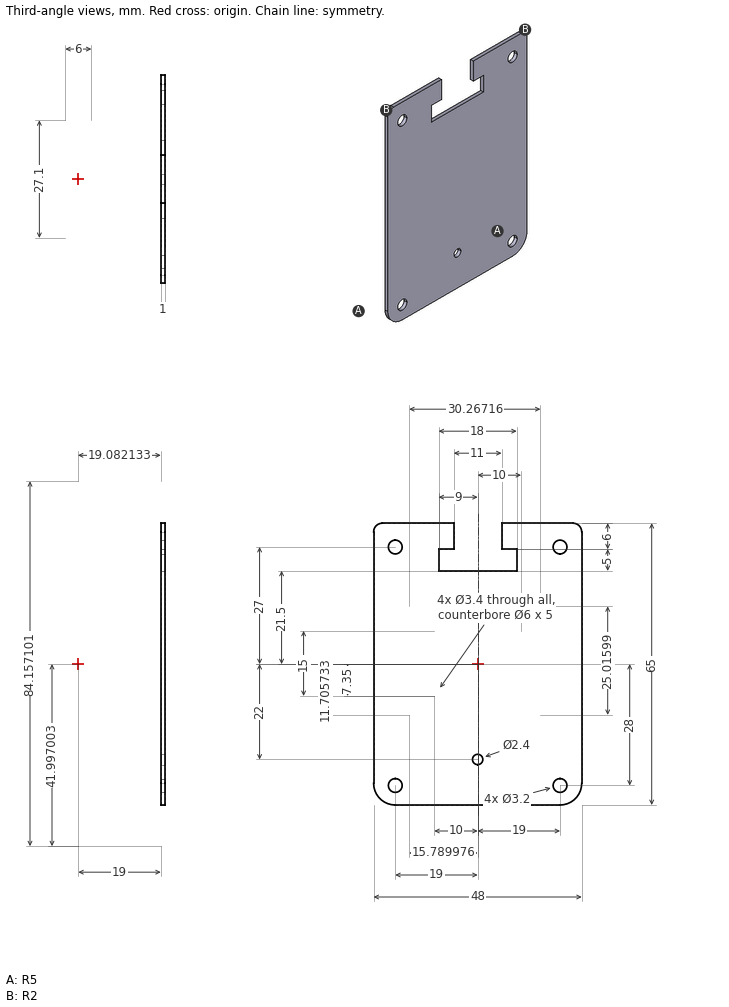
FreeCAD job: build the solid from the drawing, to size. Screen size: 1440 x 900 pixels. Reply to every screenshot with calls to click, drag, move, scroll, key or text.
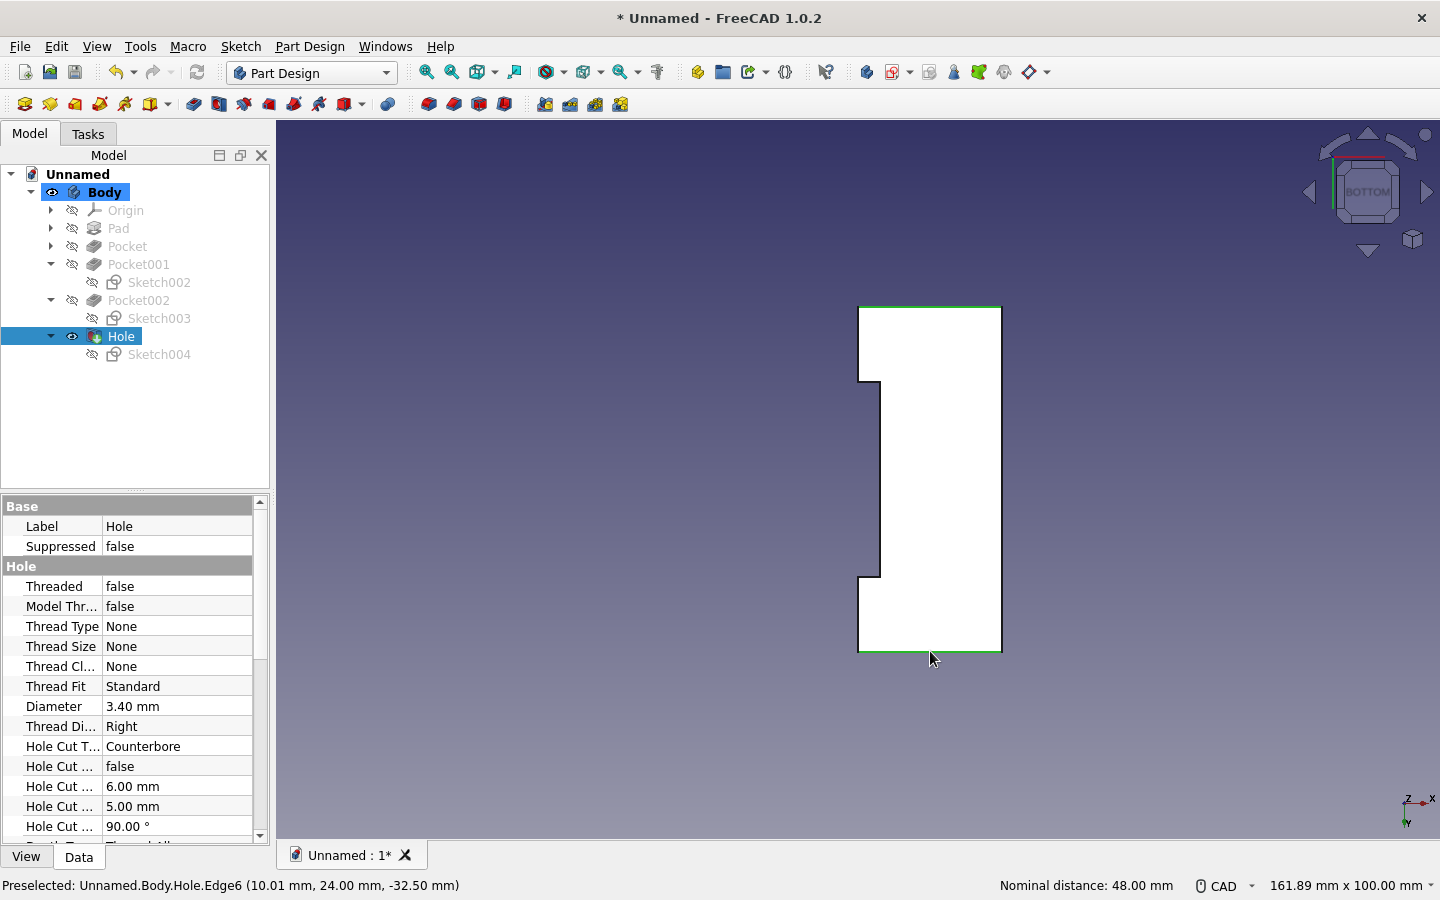
click(429, 104)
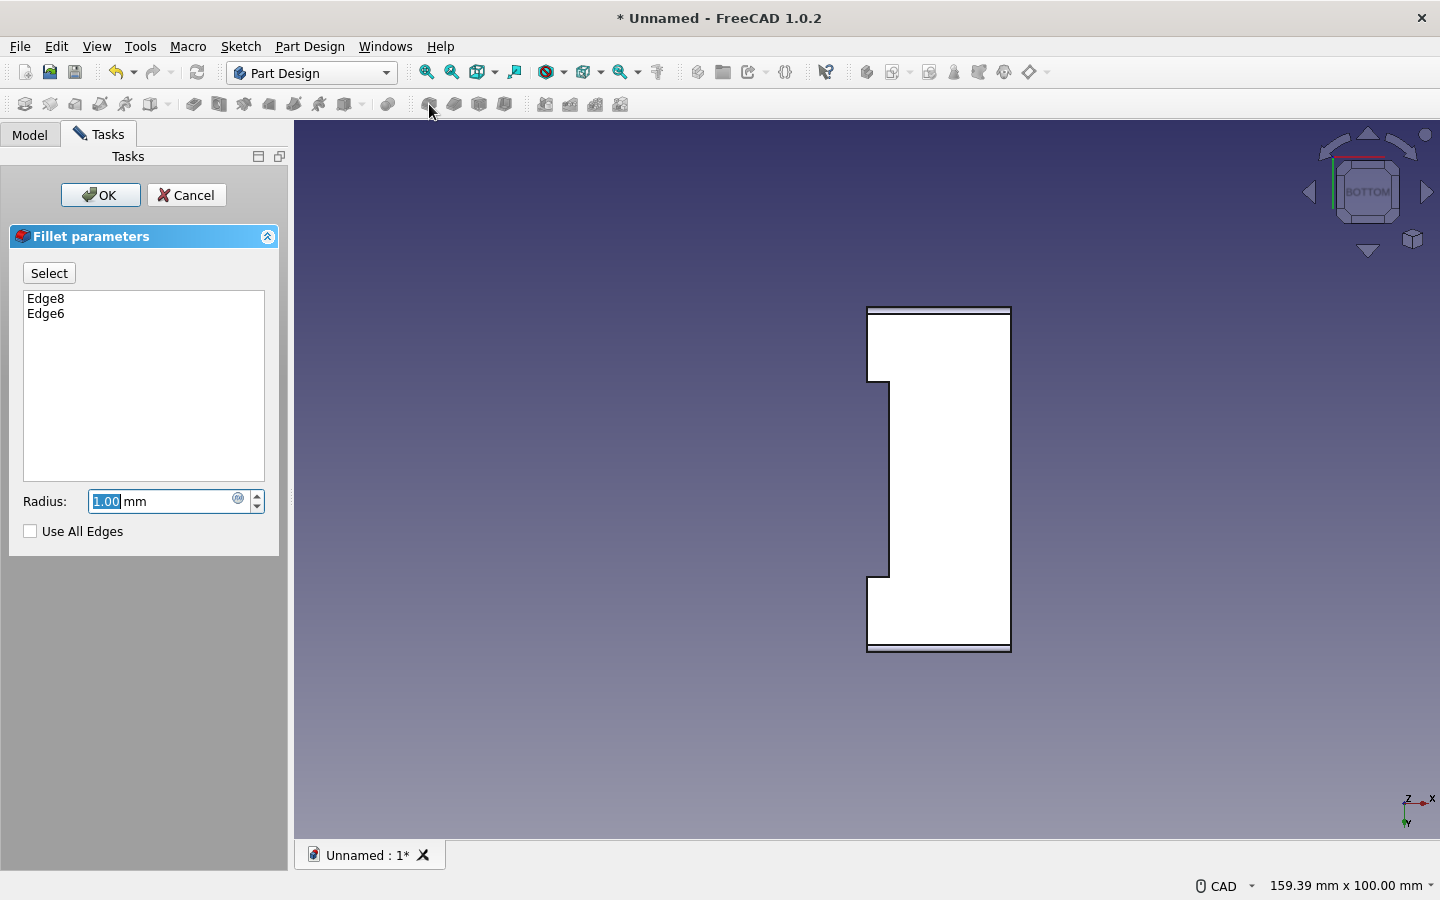
text(5)
key(Tab)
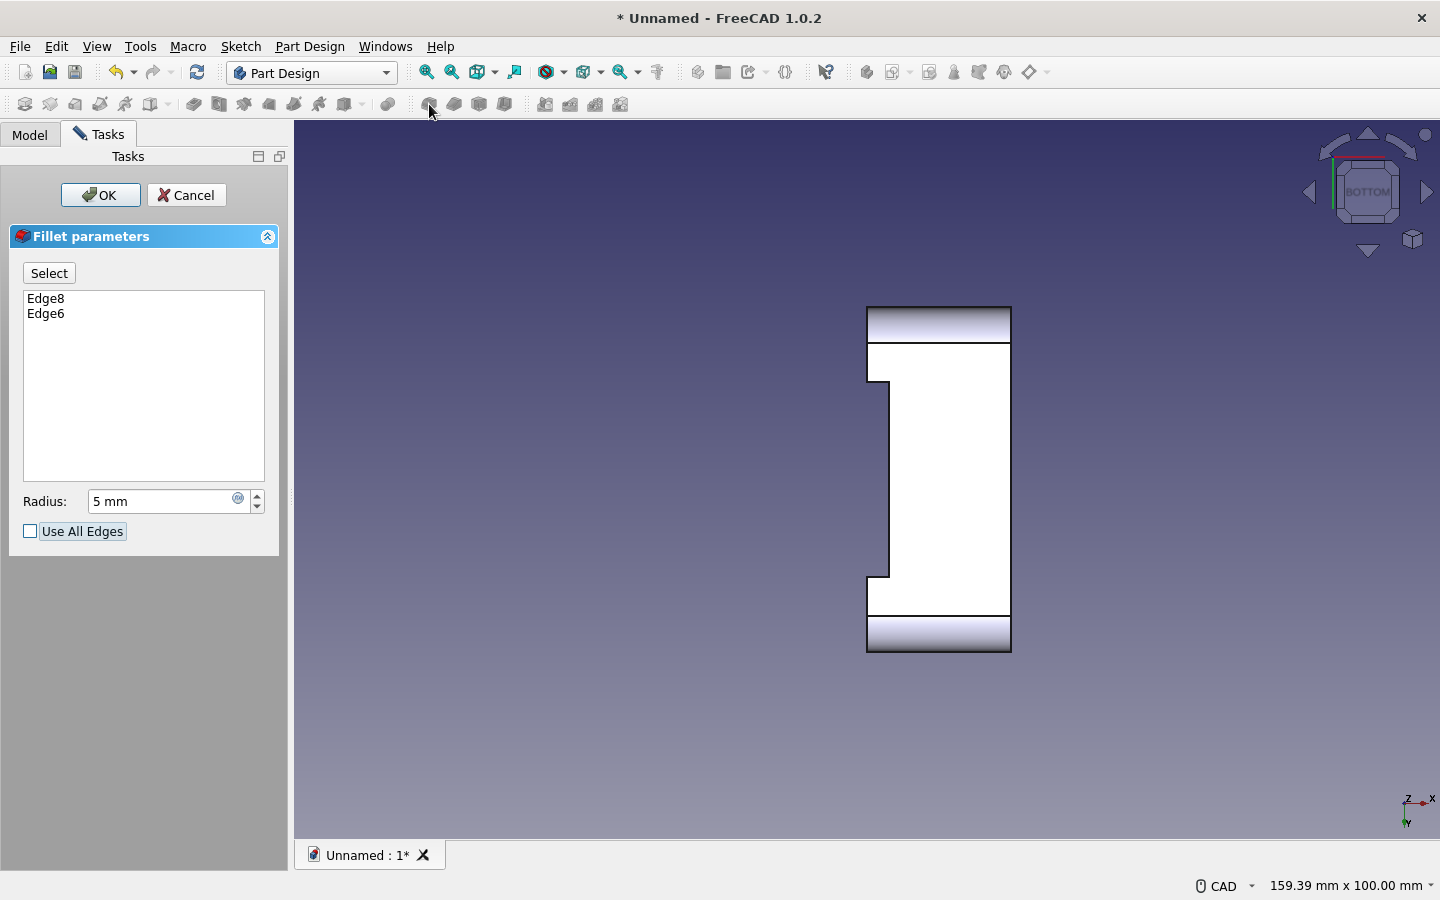
click(101, 195)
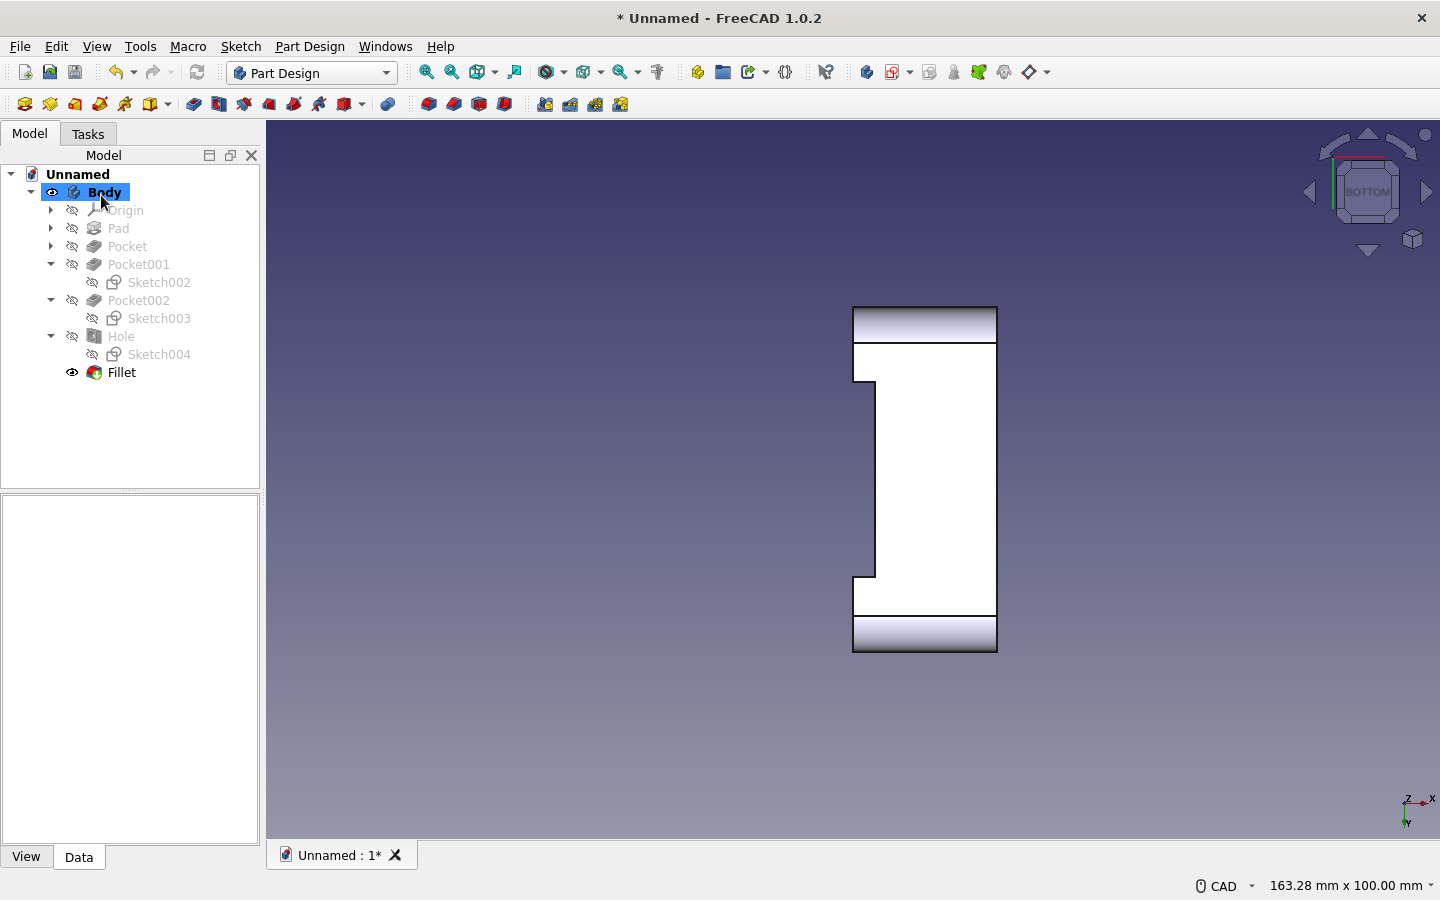
key(4)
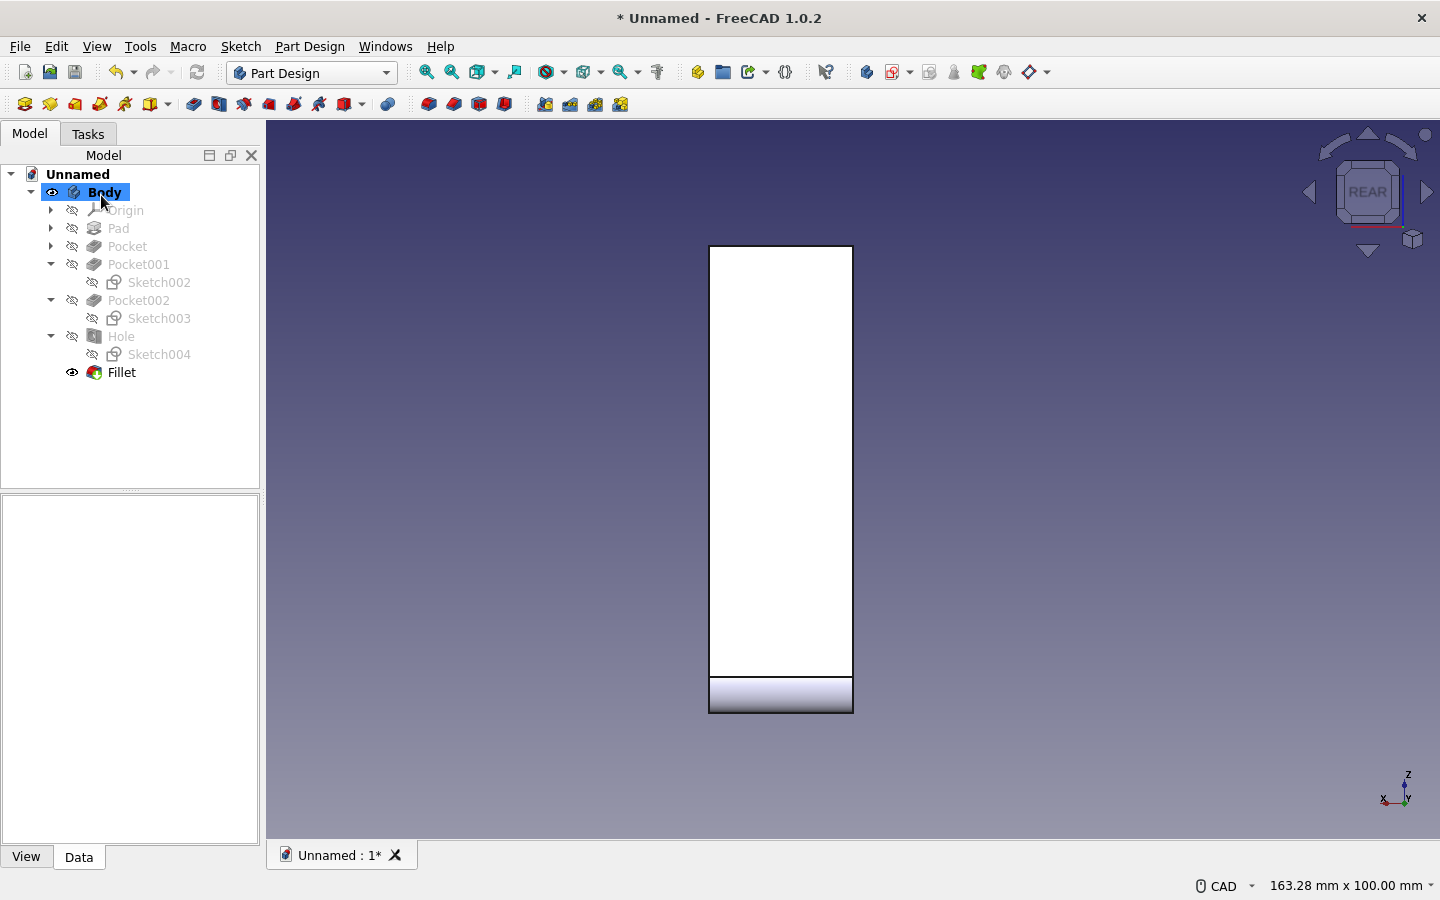
click(781, 337)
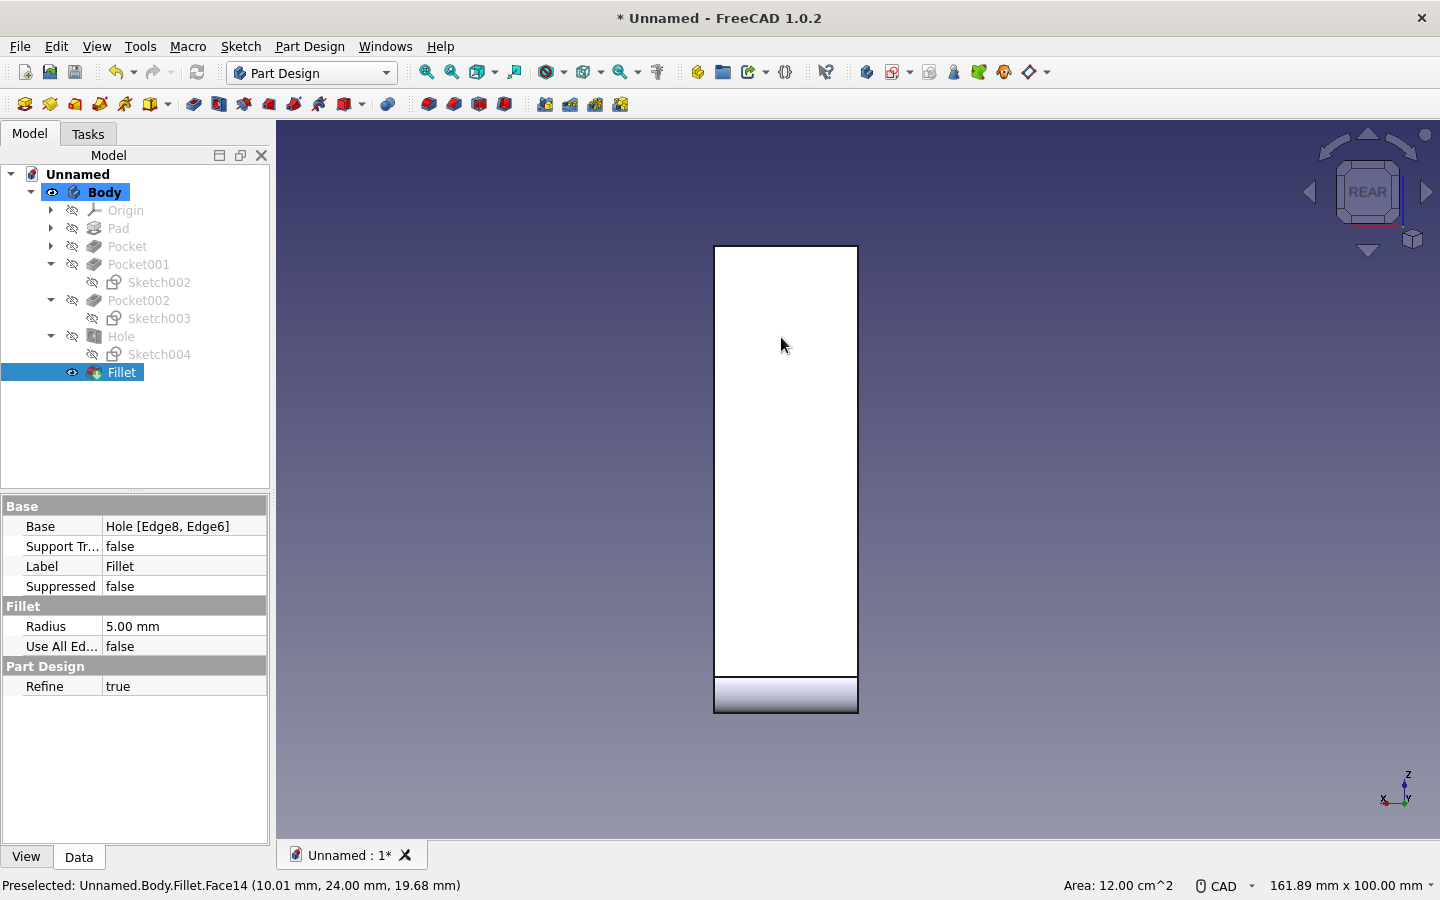
click(892, 72)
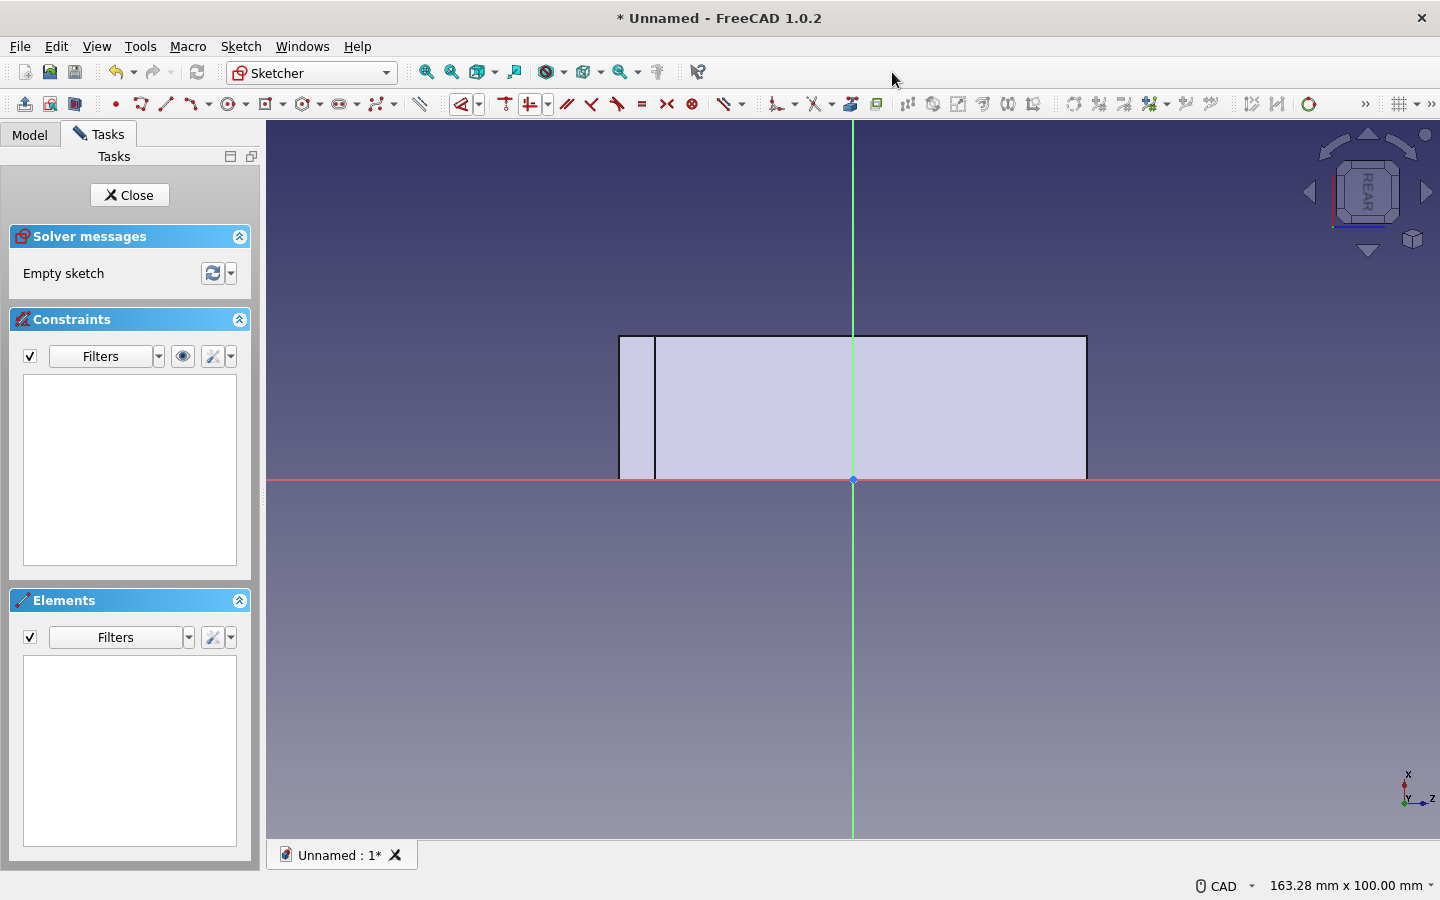
click(282, 104)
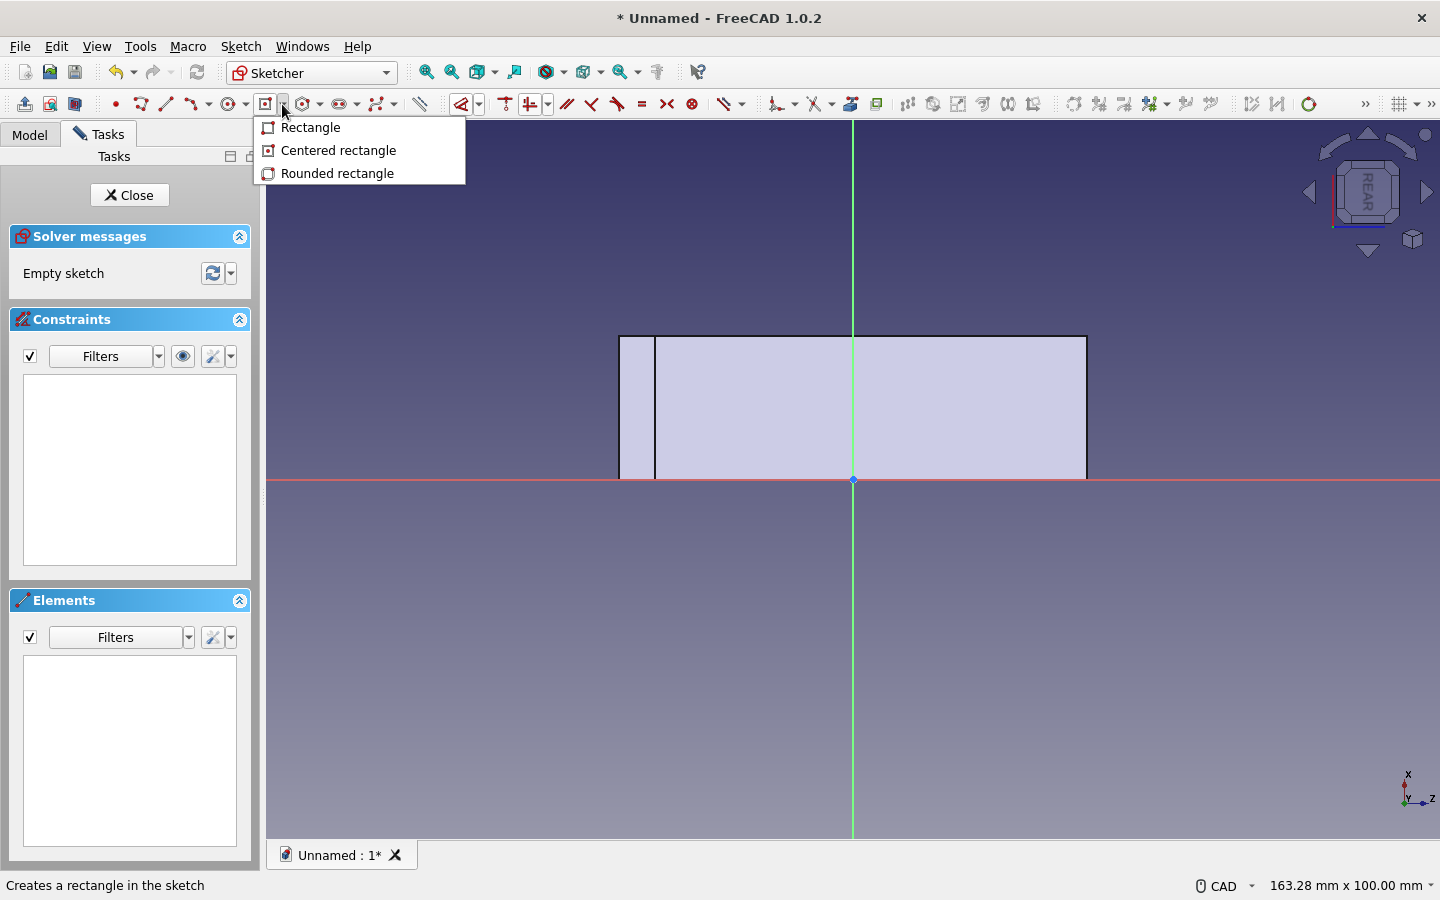
click(360, 128)